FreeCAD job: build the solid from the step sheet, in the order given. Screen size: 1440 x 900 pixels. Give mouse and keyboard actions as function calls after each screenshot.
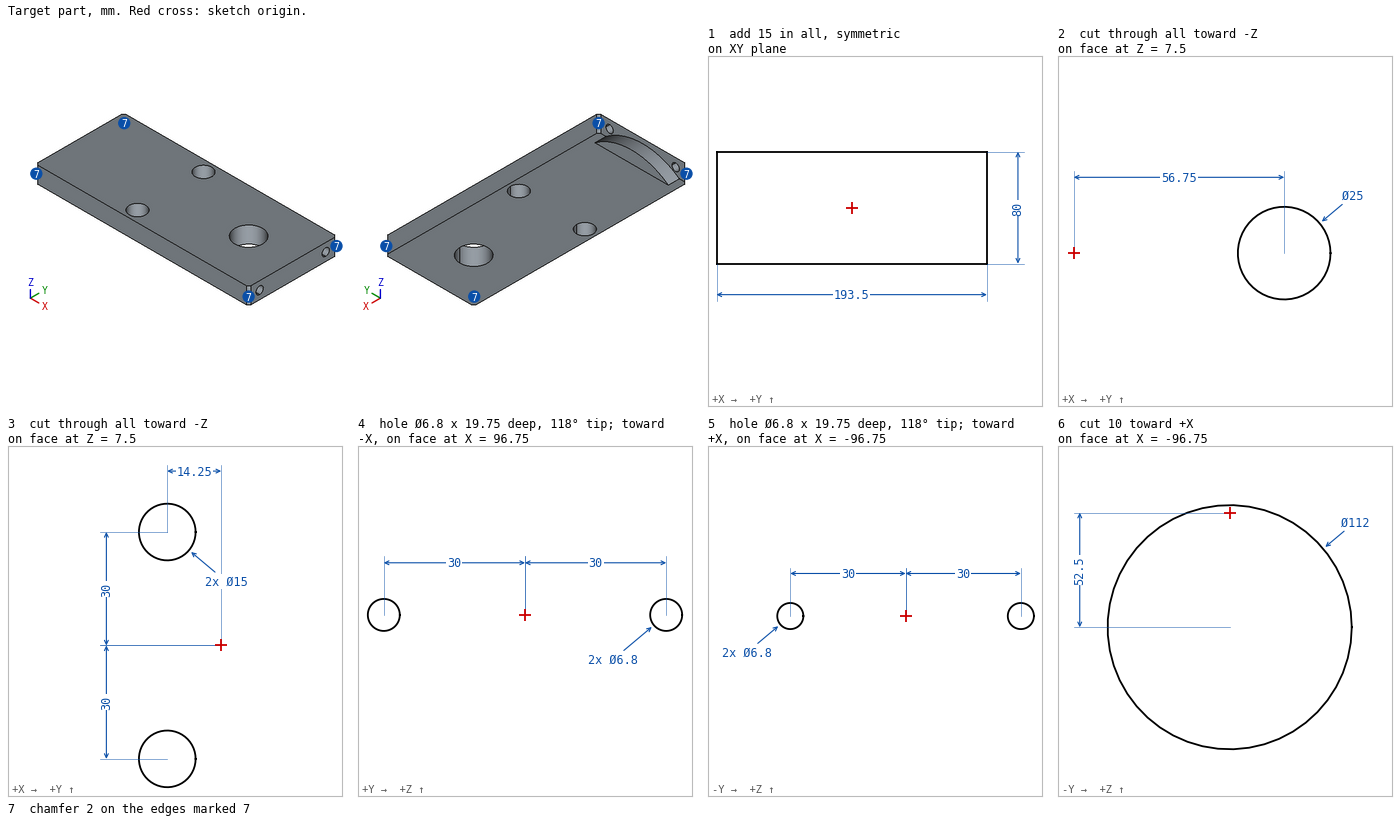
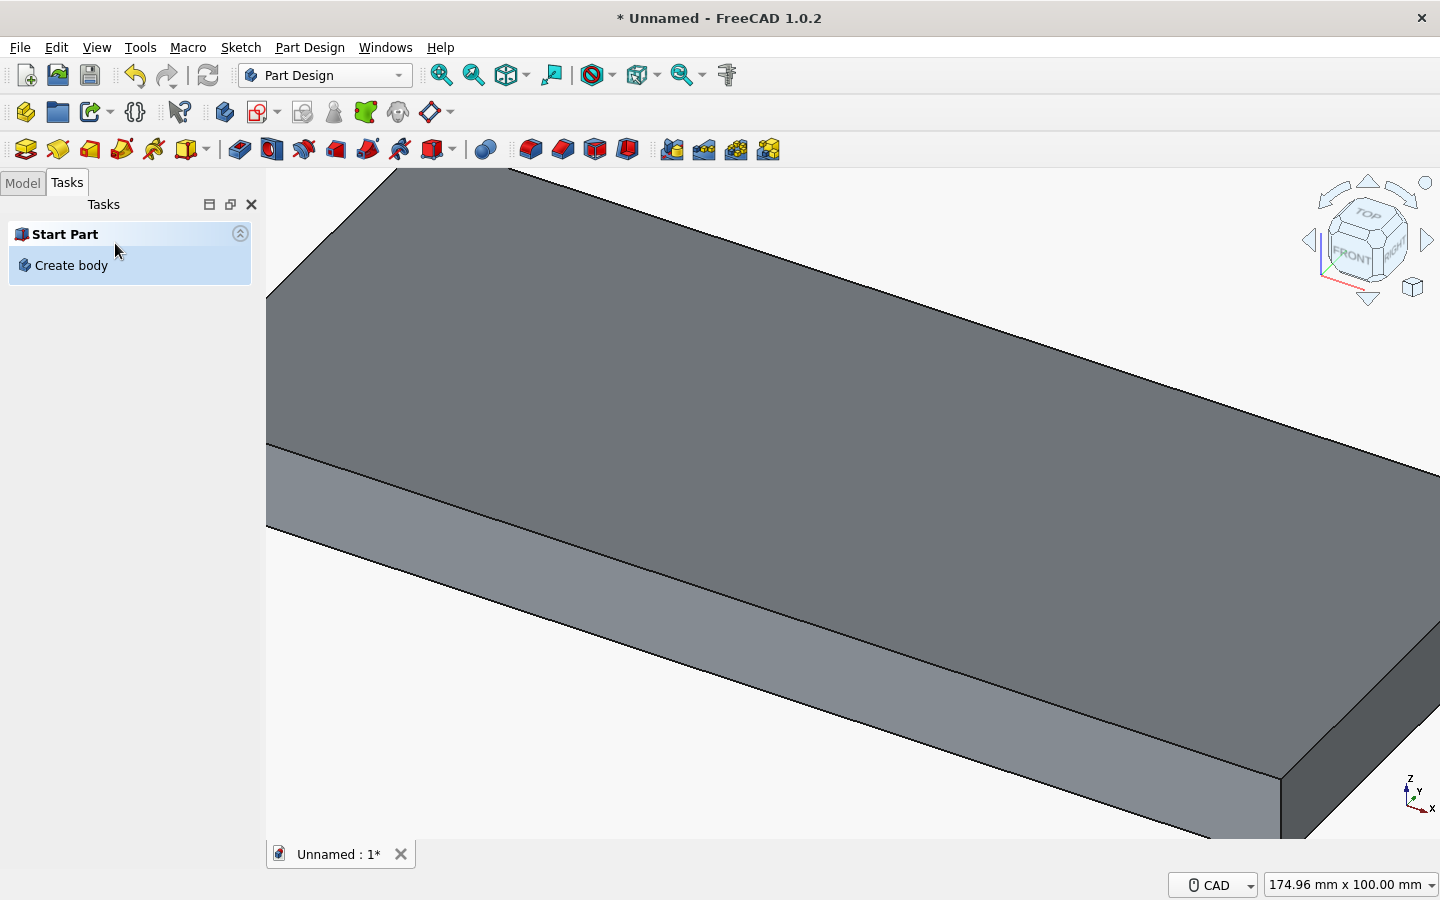
click(442, 76)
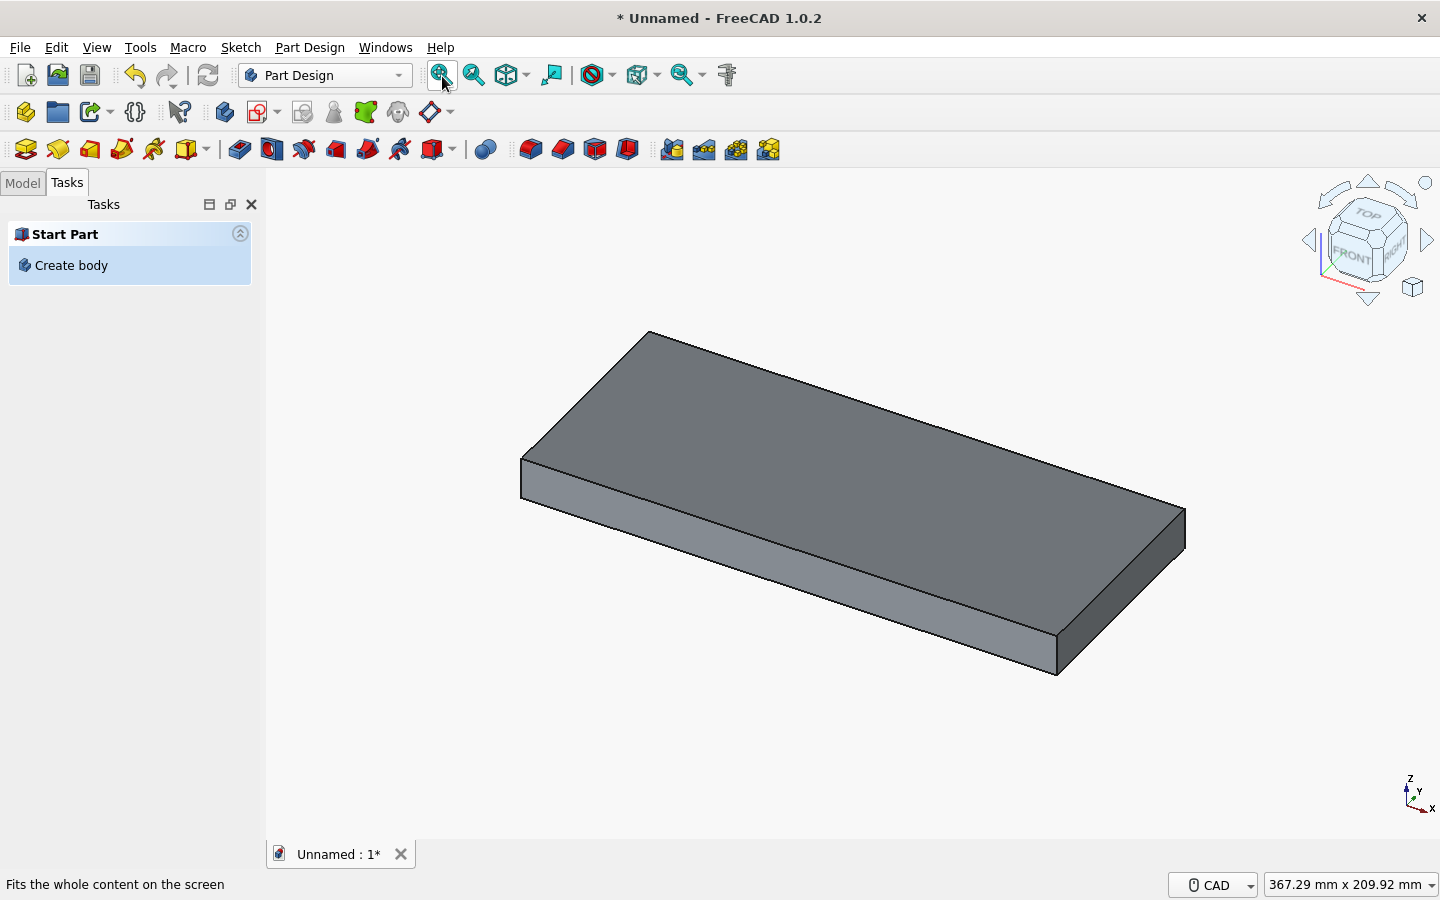
click(1006, 534)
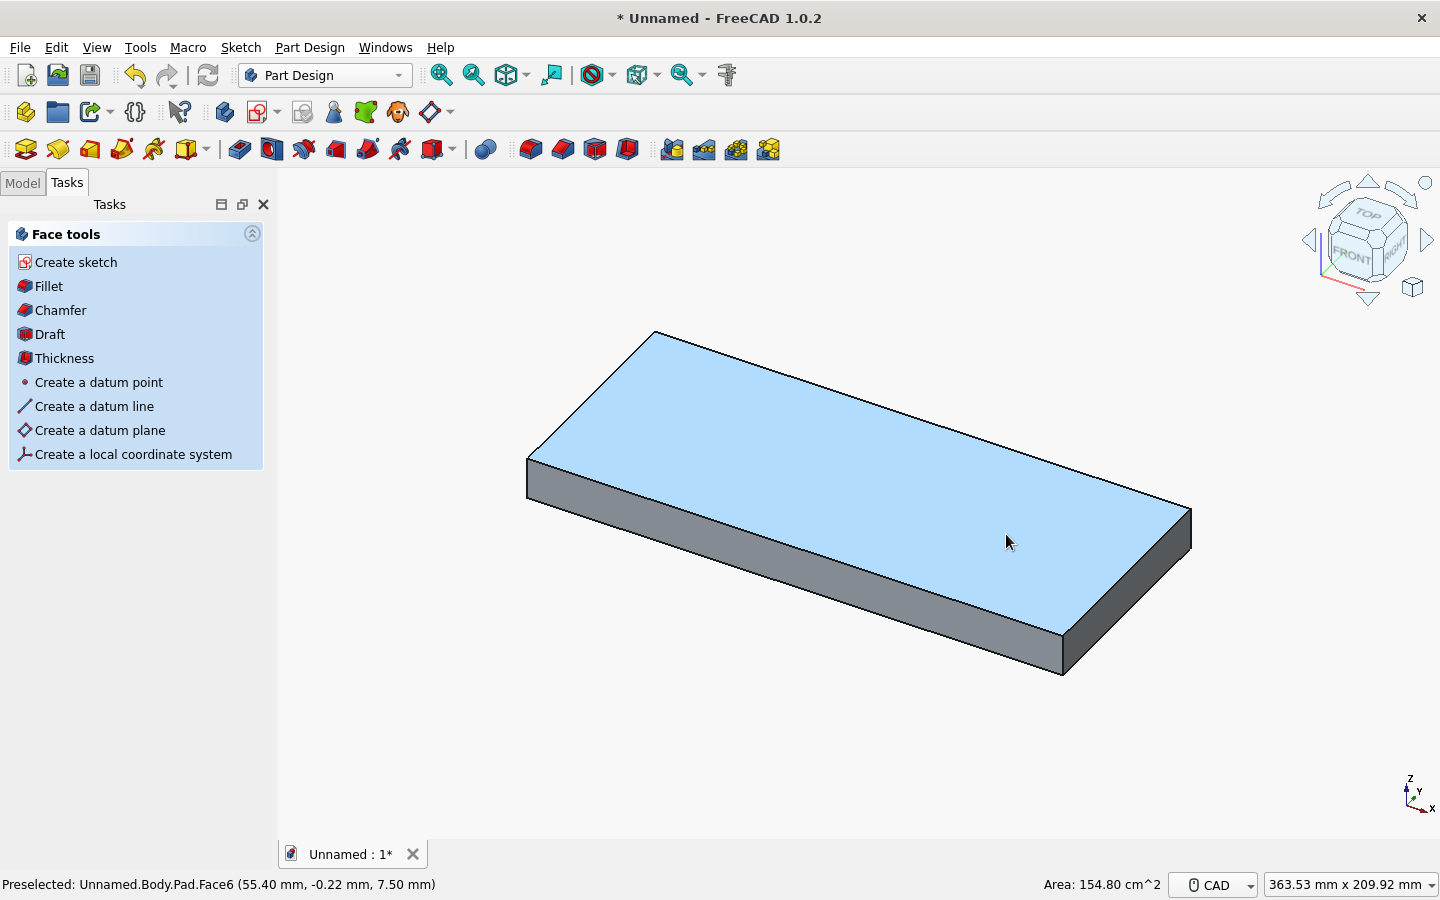
click(258, 112)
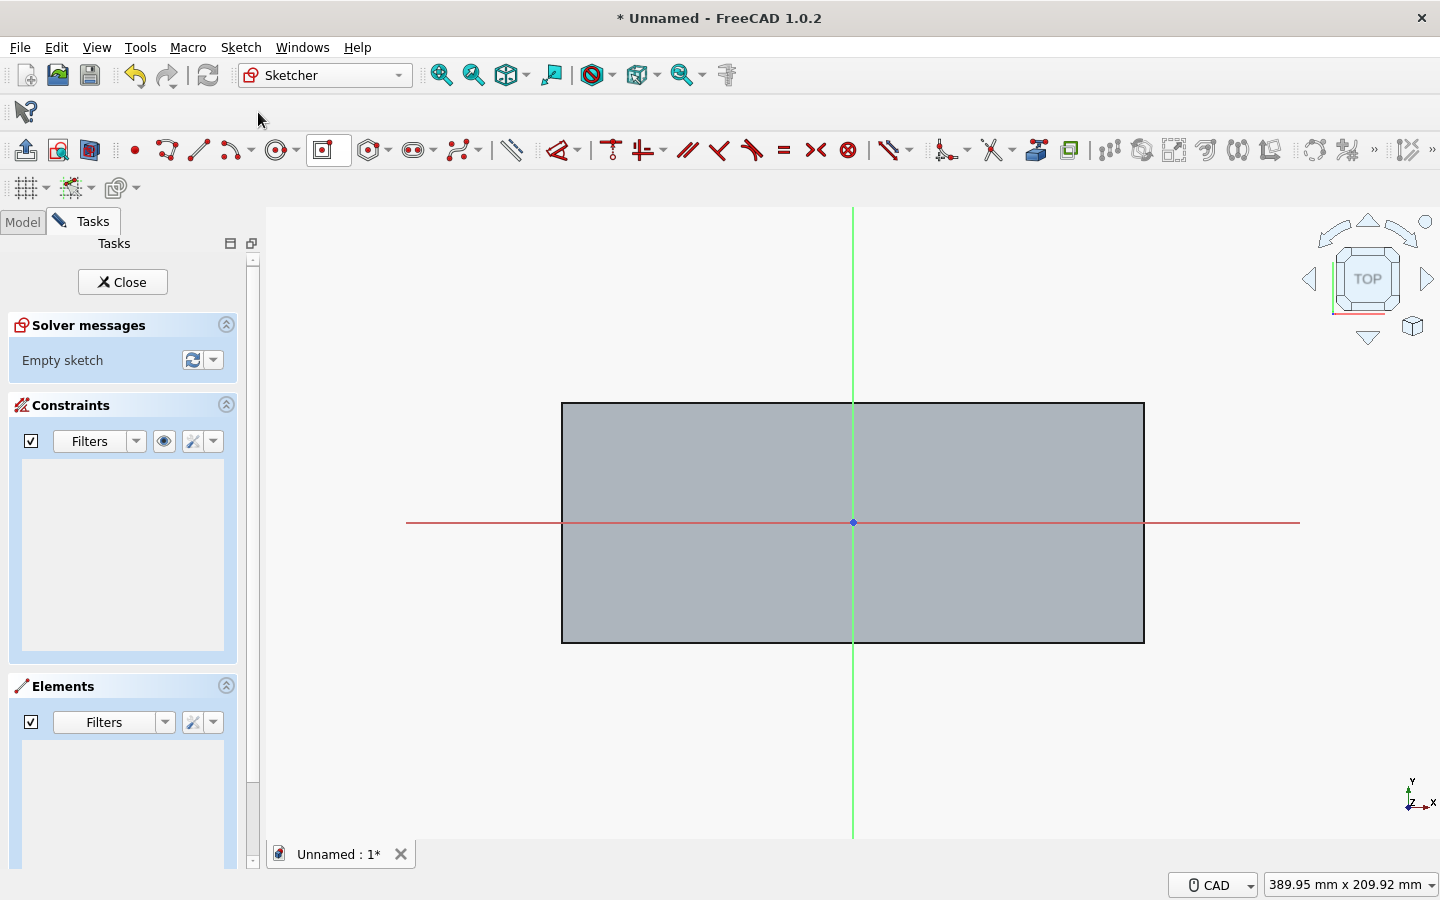
scroll(1084, 523, up, 8)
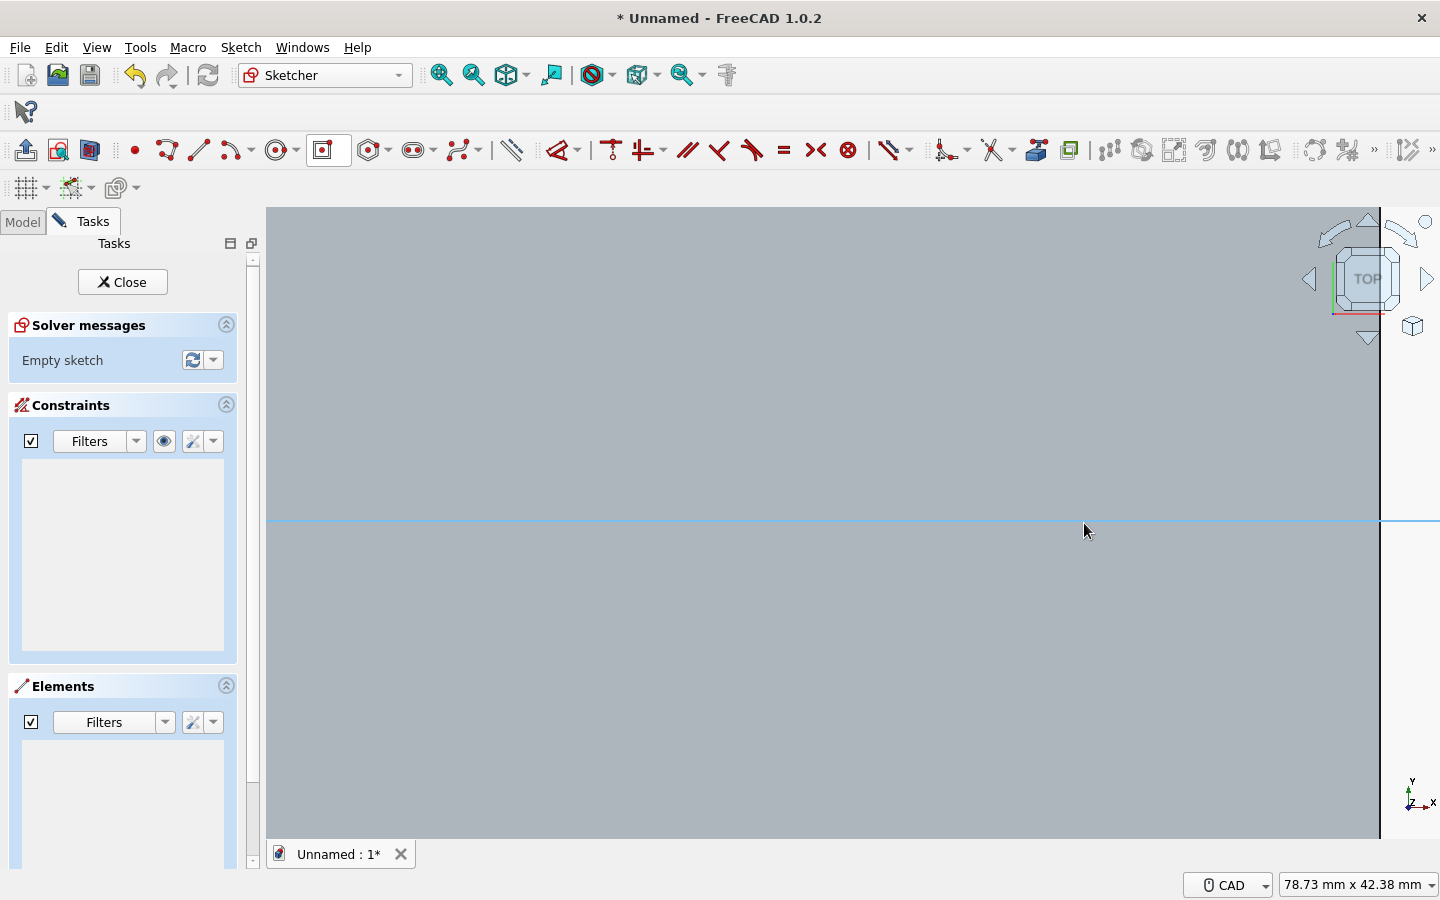
click(276, 150)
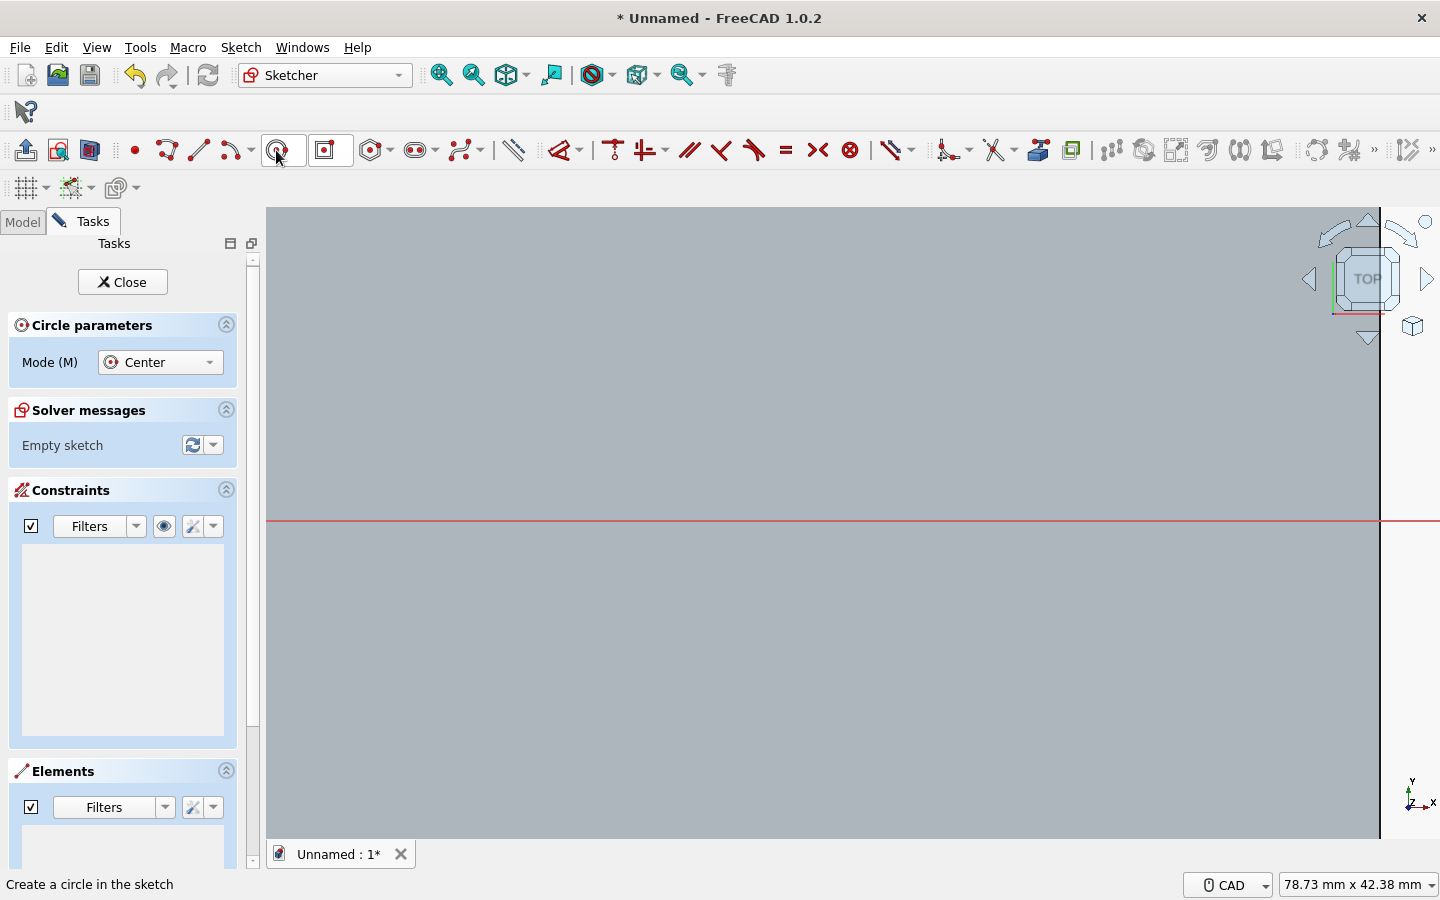
click(783, 521)
move(915, 389)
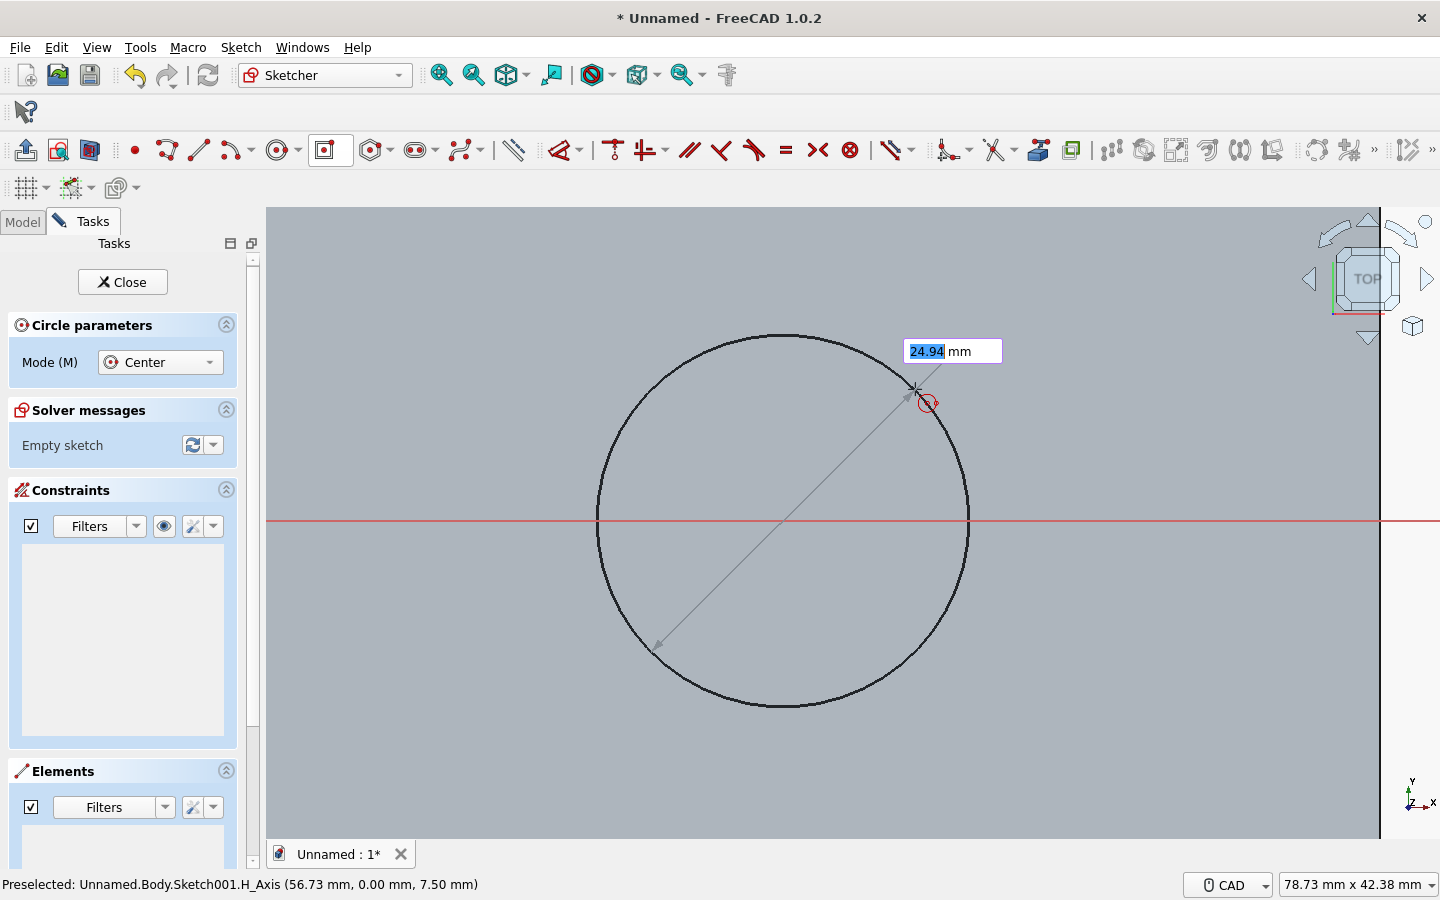
text(25)
key(Return)
key(Escape)